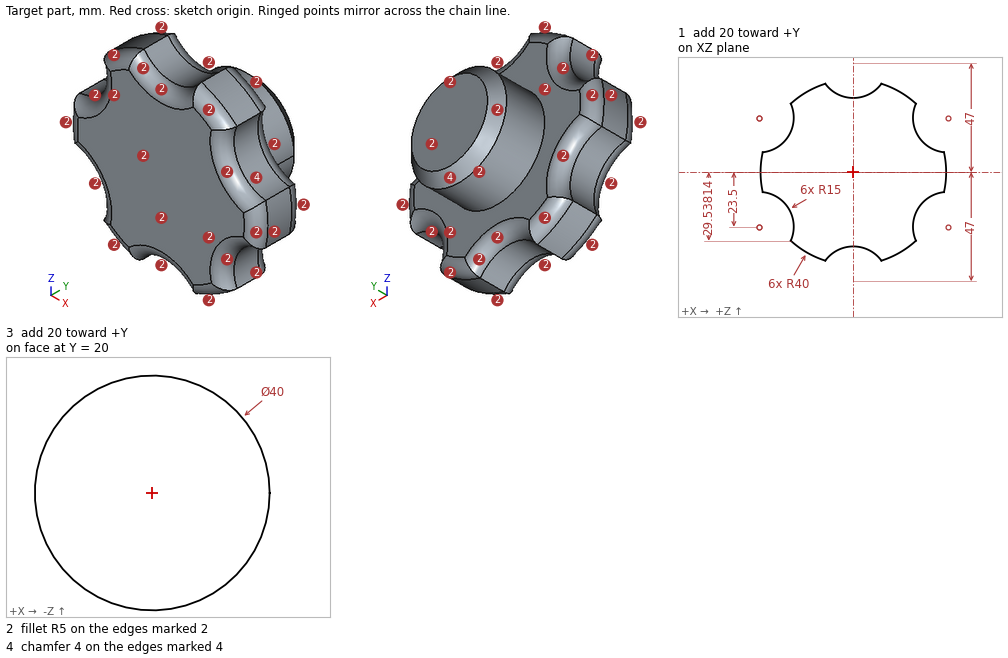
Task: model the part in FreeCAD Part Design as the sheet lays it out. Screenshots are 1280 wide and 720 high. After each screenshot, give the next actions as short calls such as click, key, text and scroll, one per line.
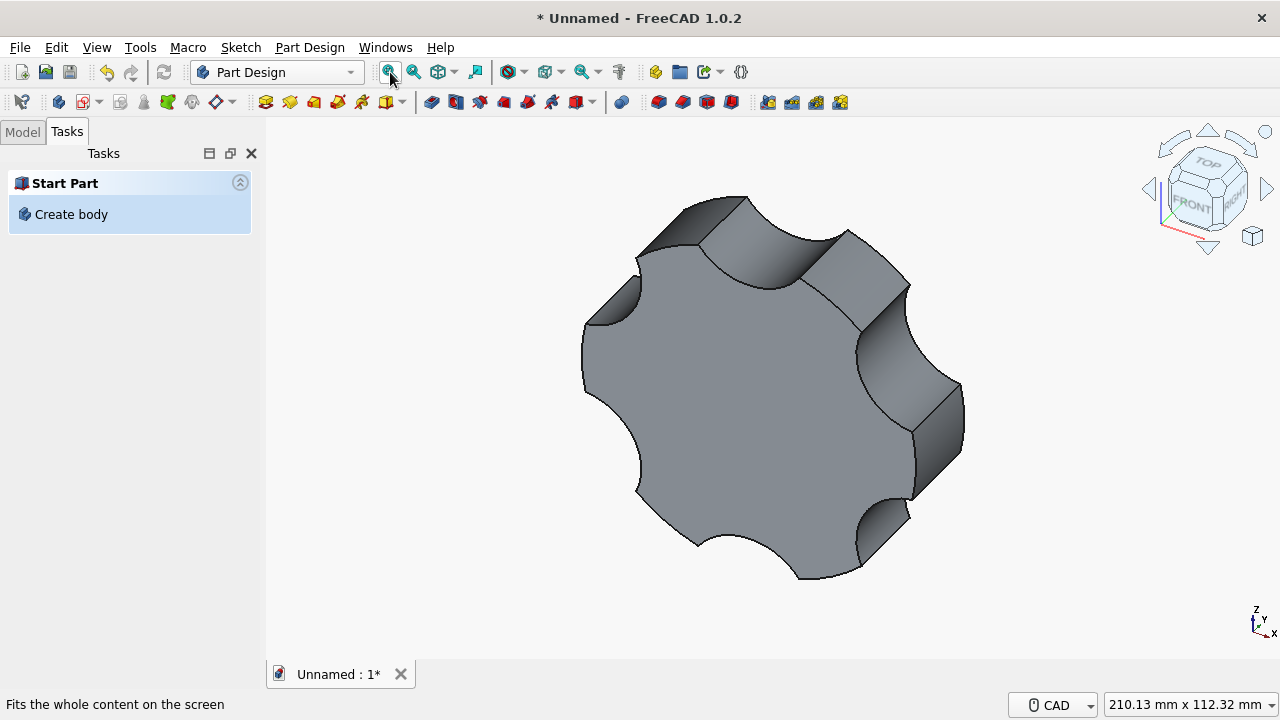
click(749, 411)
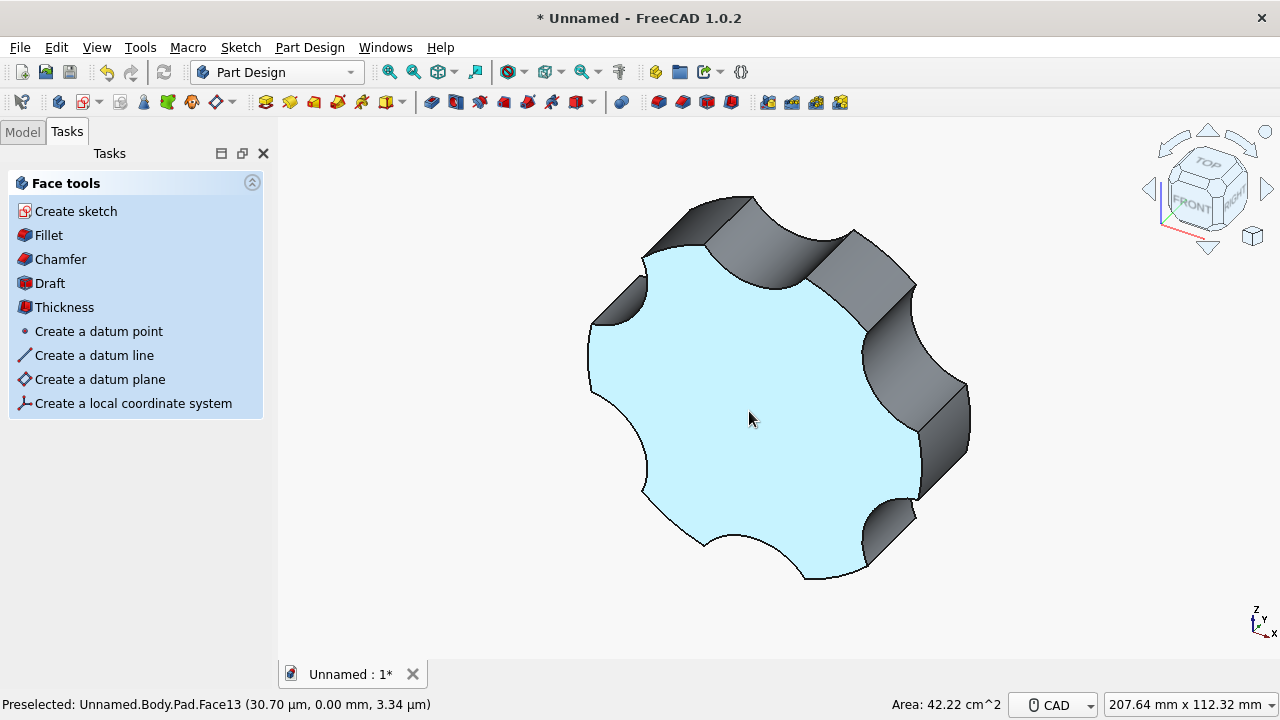
key(0)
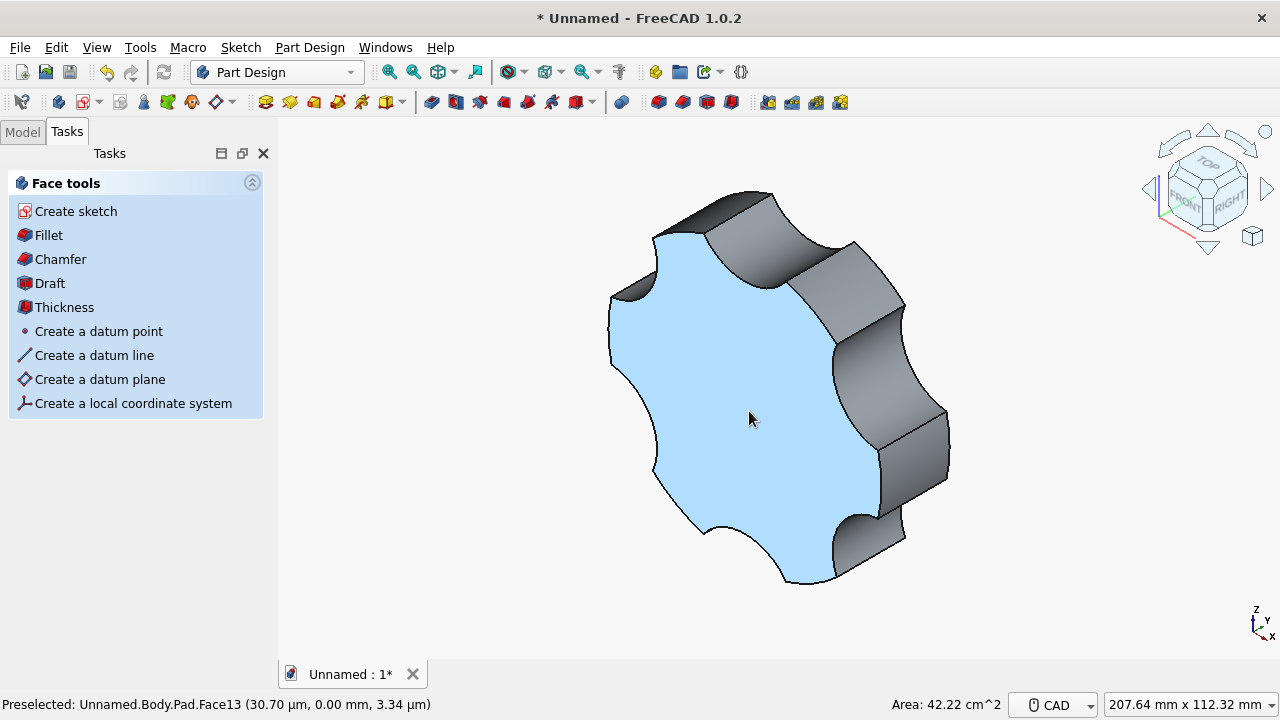
key(2)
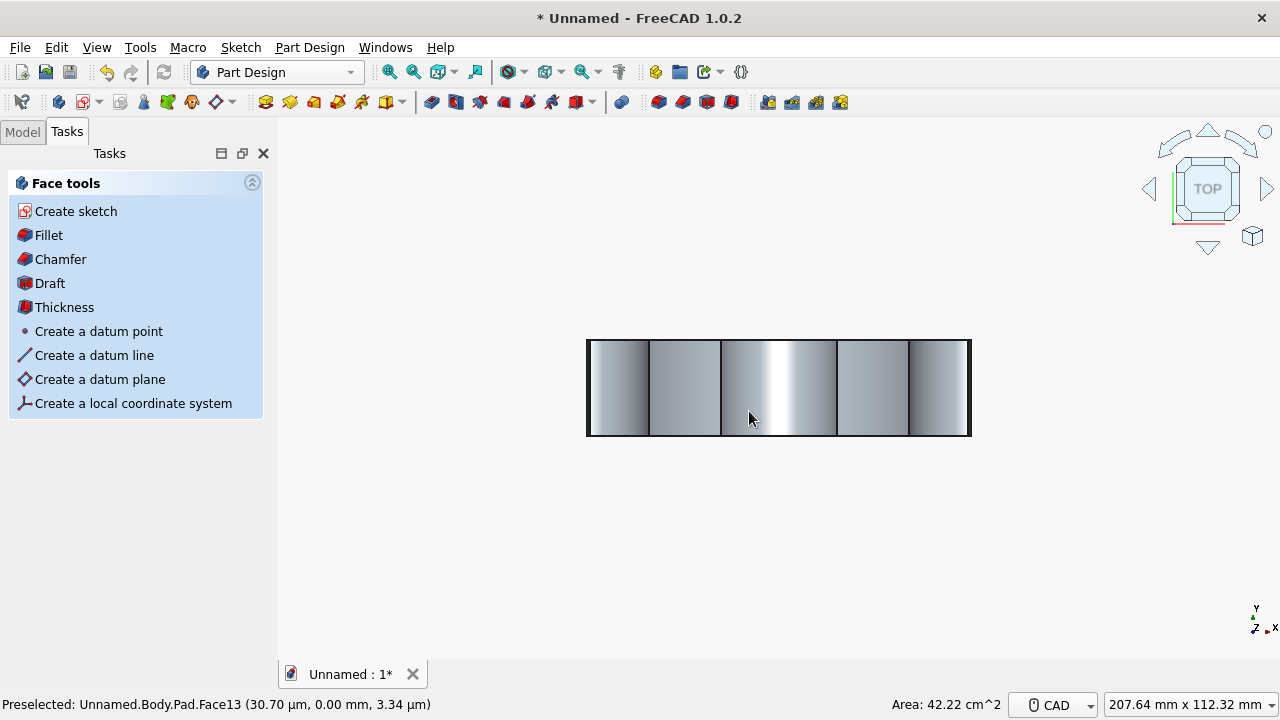
click(390, 72)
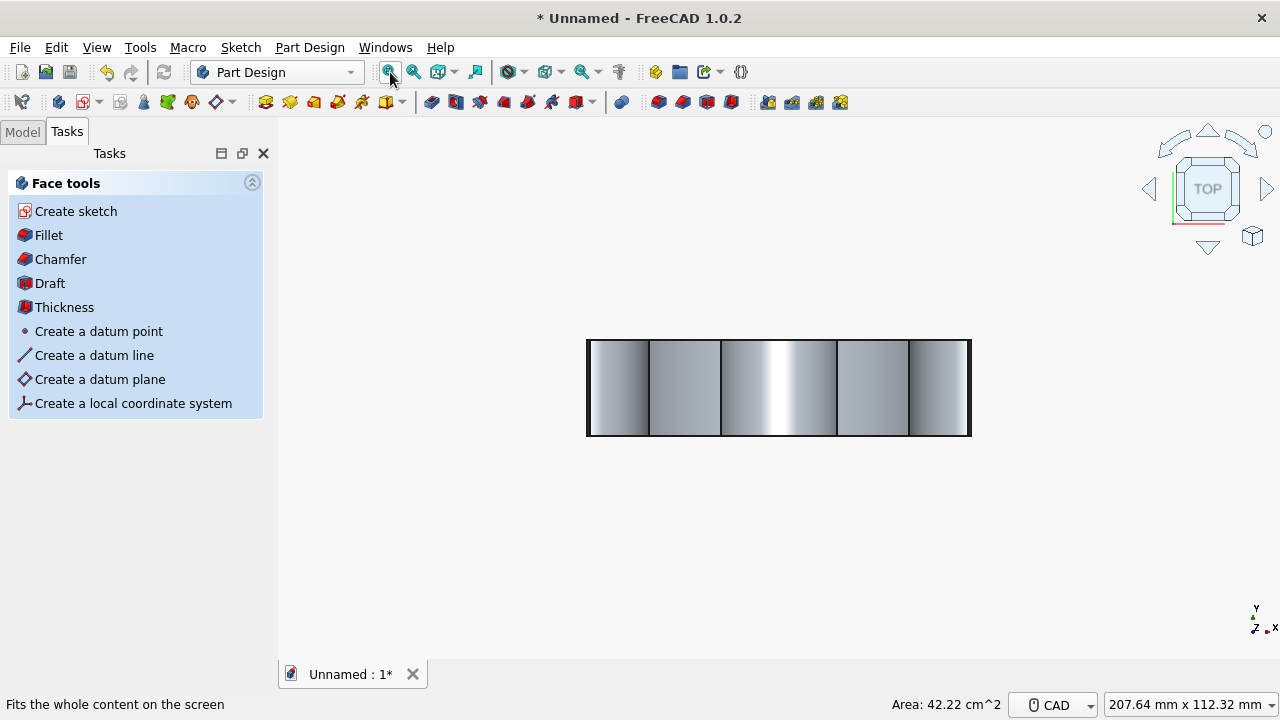
key(1)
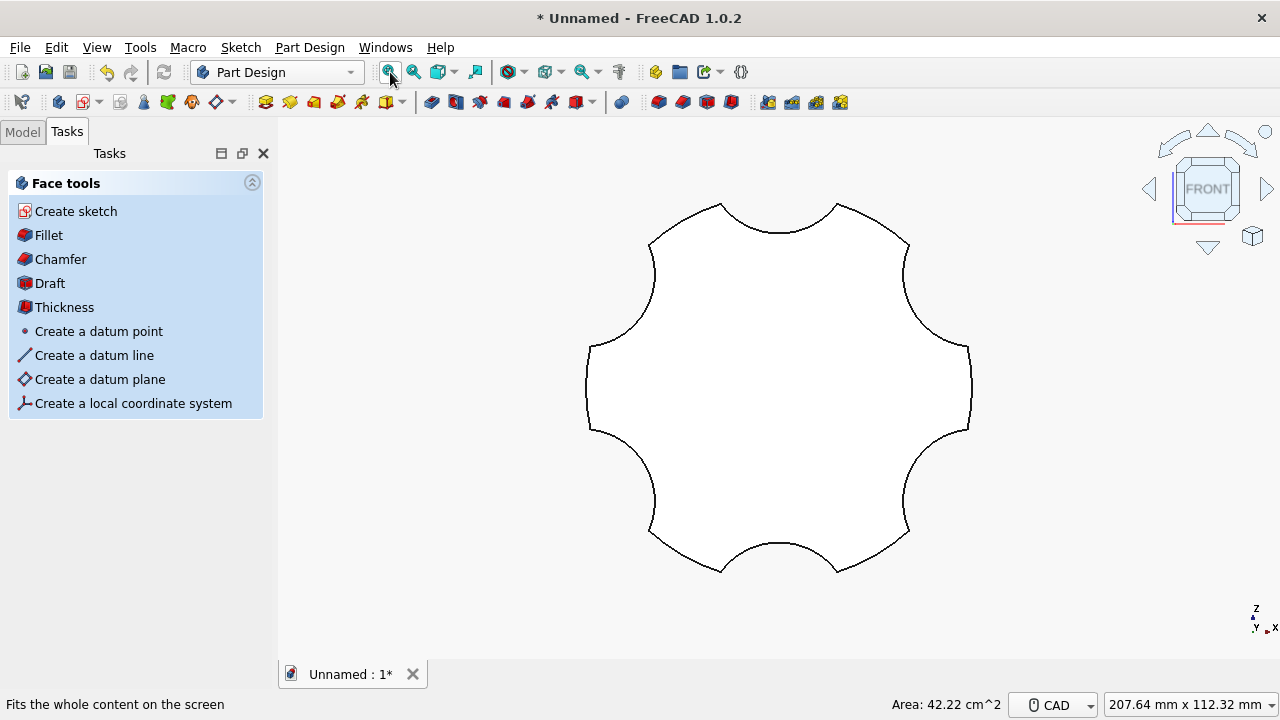
key(3)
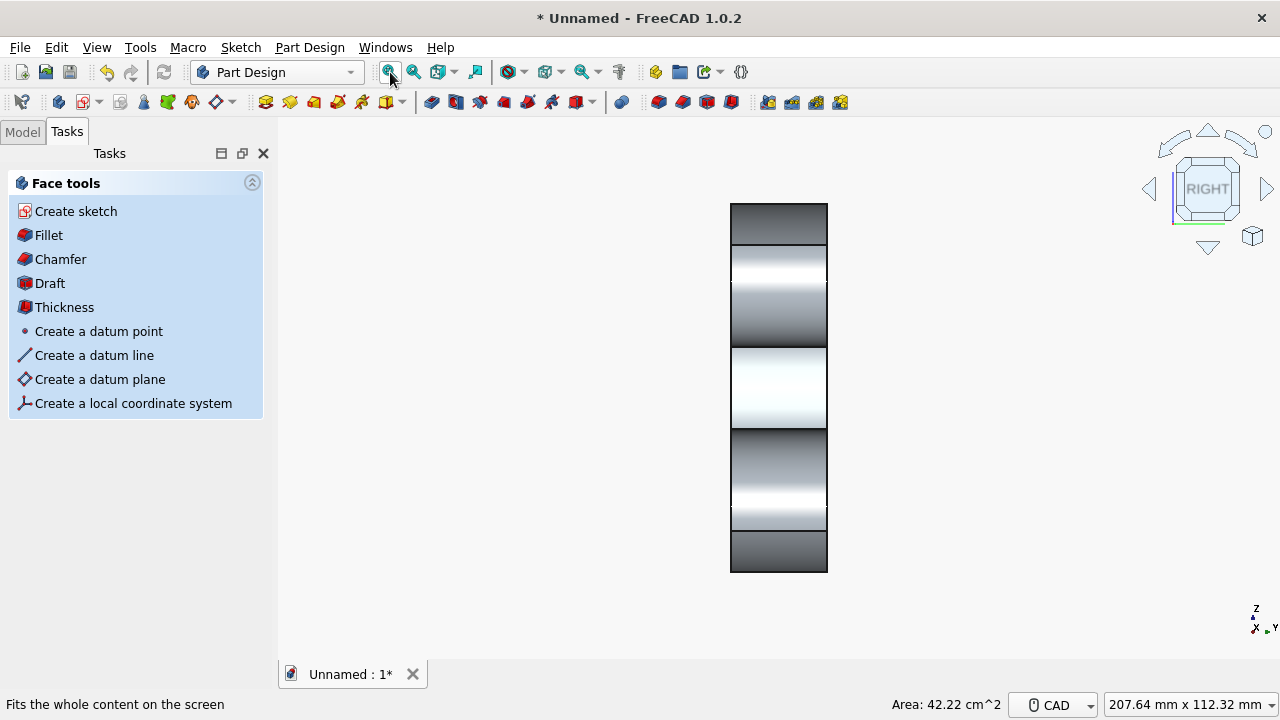
key(5)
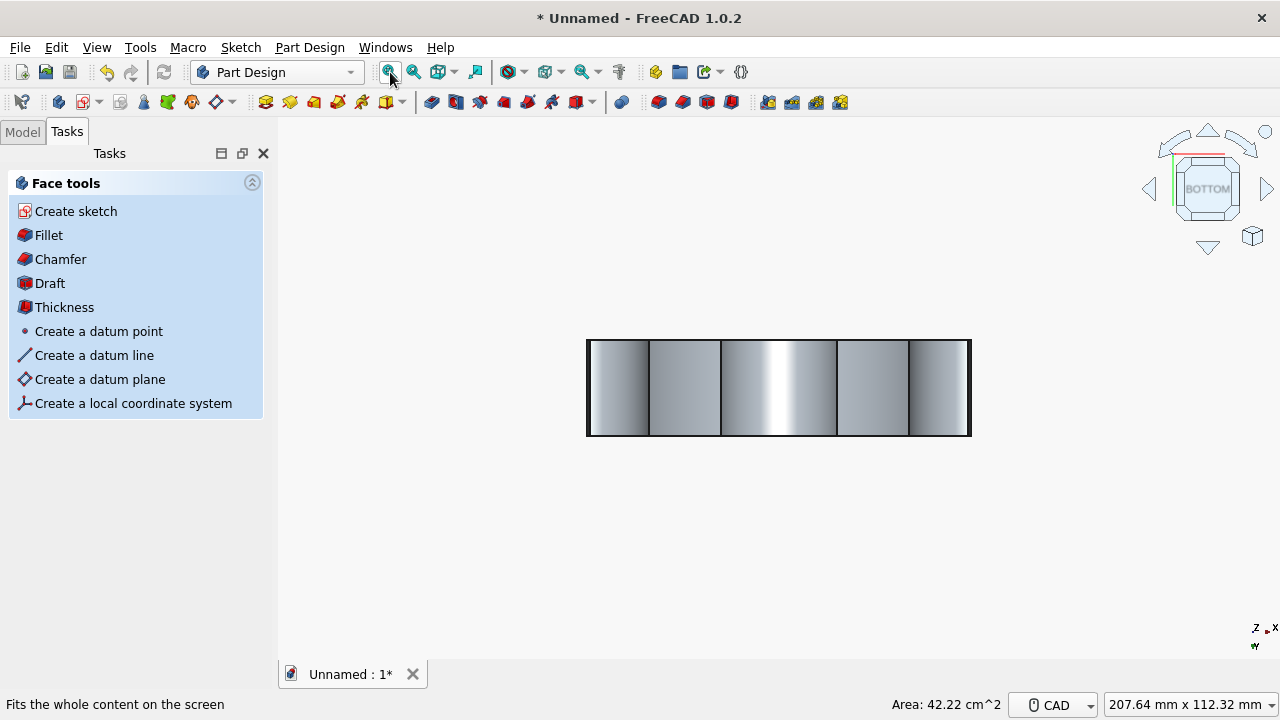
click(390, 72)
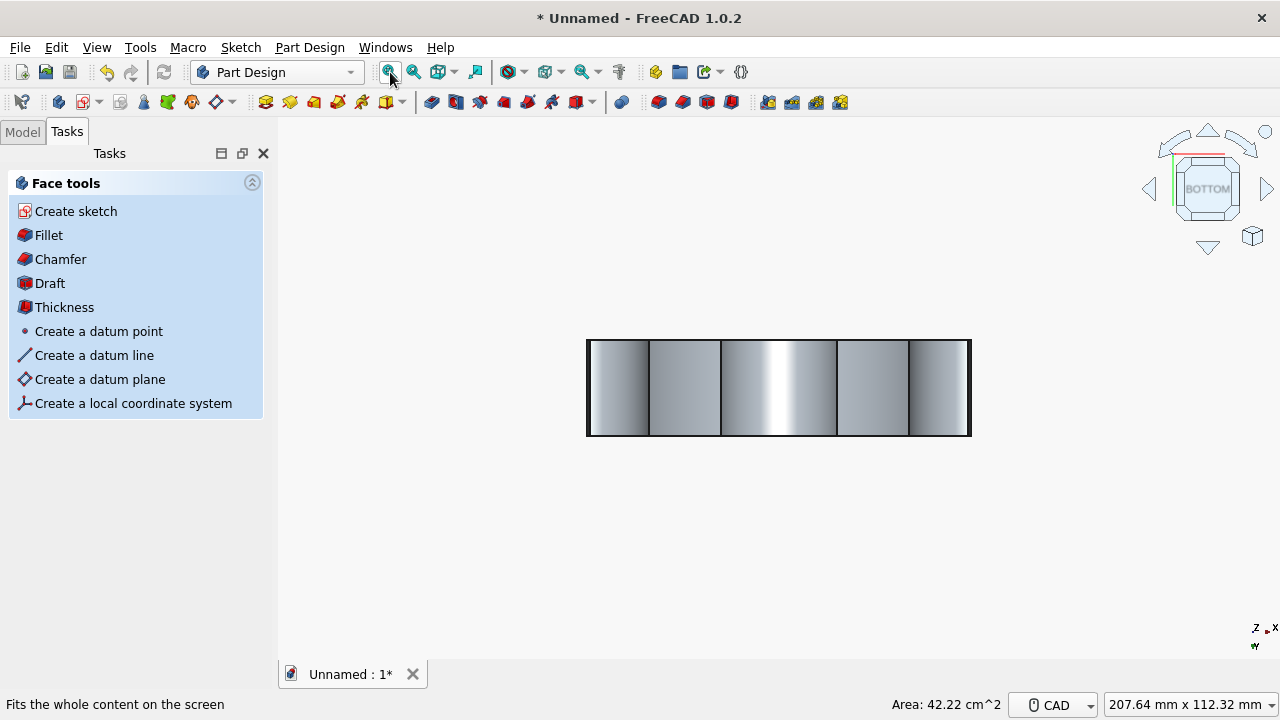
key(4)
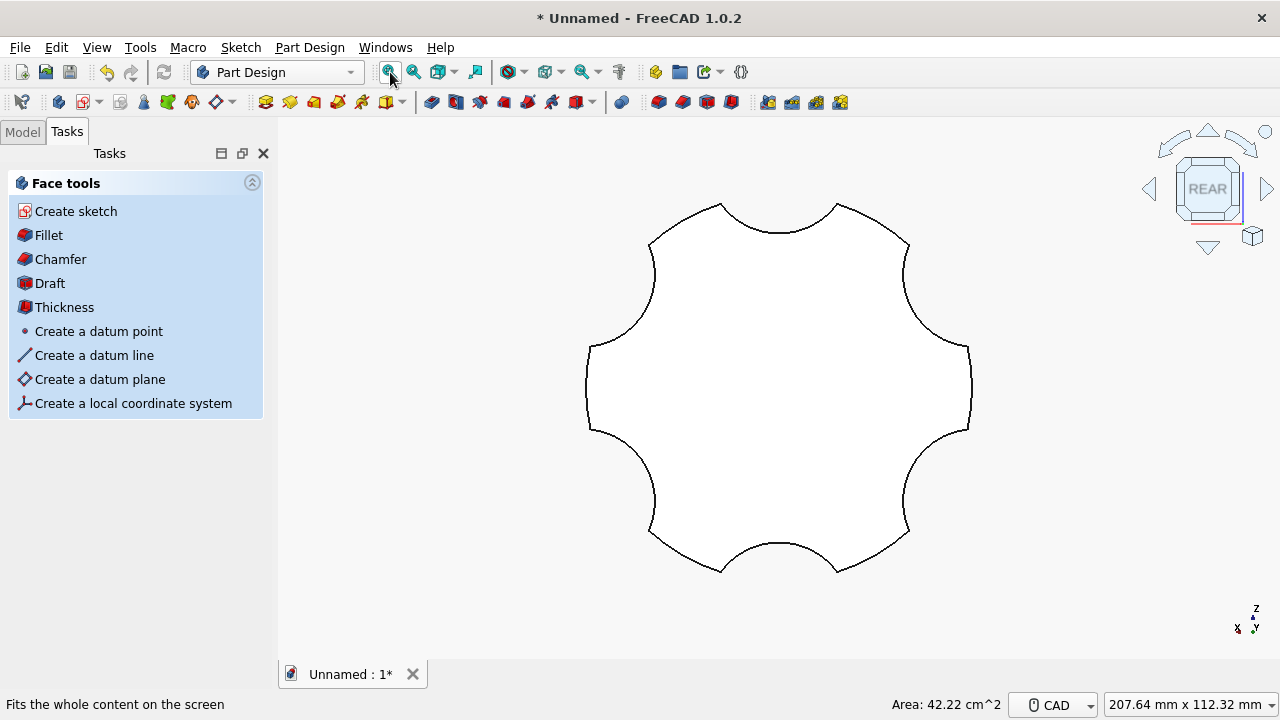
click(779, 387, ctrl)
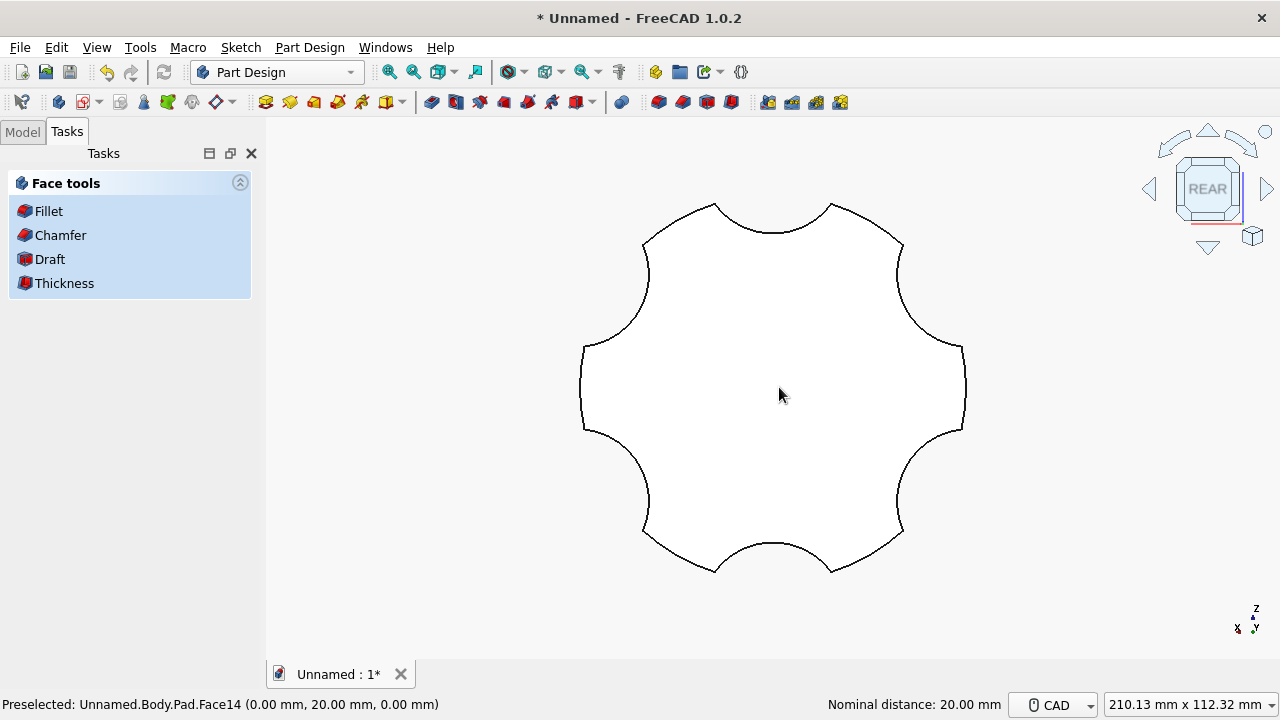
click(660, 102)